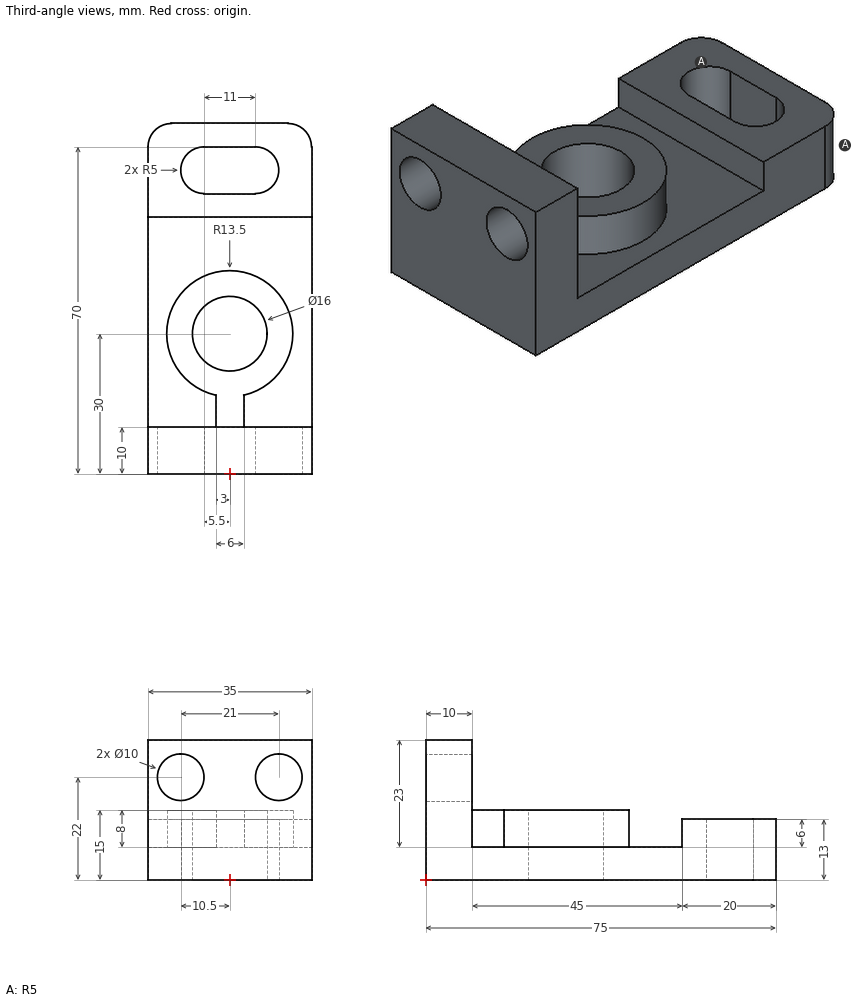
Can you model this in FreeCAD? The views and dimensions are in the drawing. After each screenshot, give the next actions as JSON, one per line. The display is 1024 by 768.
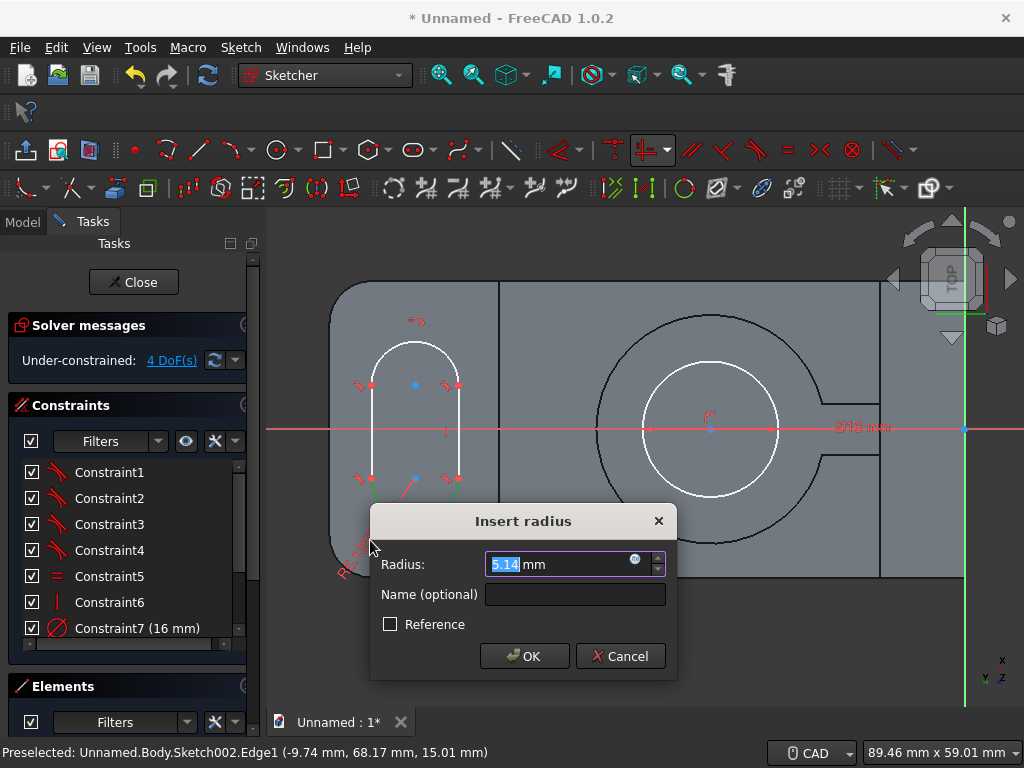
{"action": "type", "text": "5"}
{"action": "key", "text": "Return"}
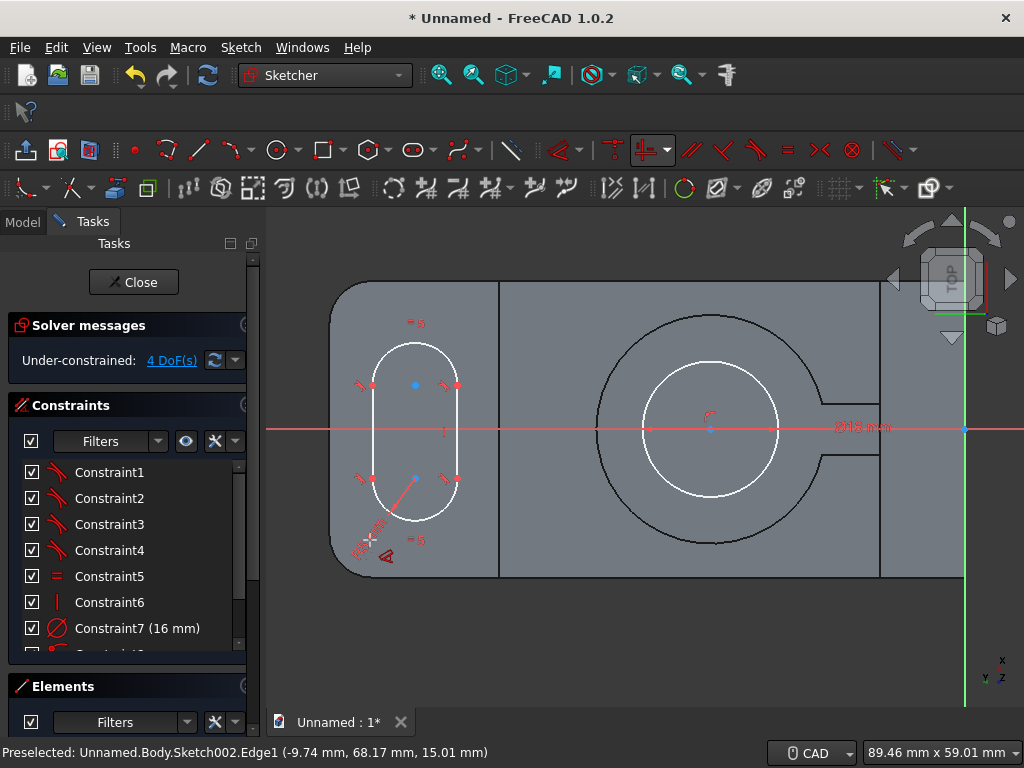
{"action": "left_click", "coordinate": [373, 450]}
{"action": "left_click", "coordinate": [339, 410]}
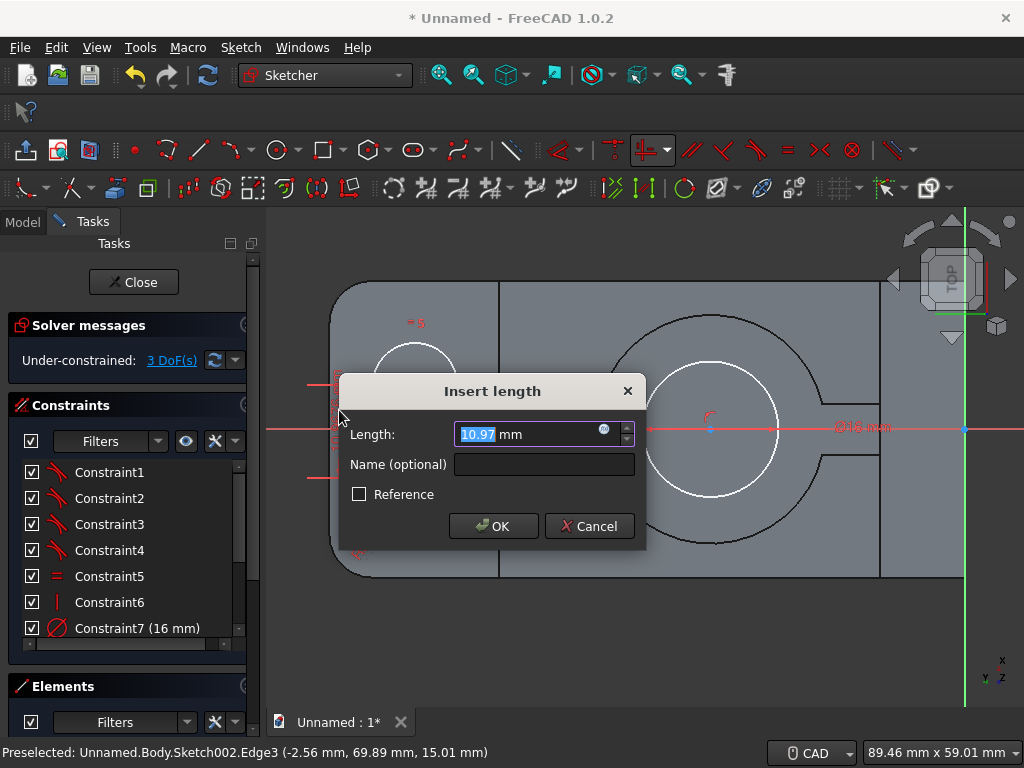
{"action": "type", "text": "11"}
{"action": "key", "text": "Return"}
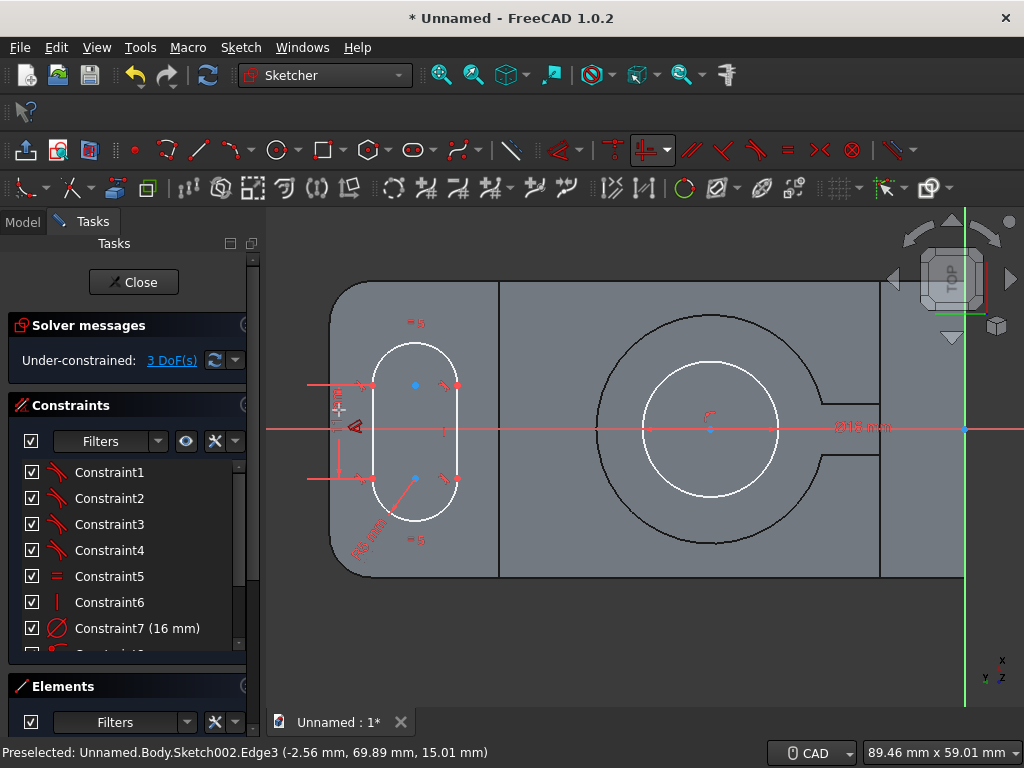
{"action": "left_click", "coordinate": [711, 429]}
{"action": "left_click", "coordinate": [785, 463]}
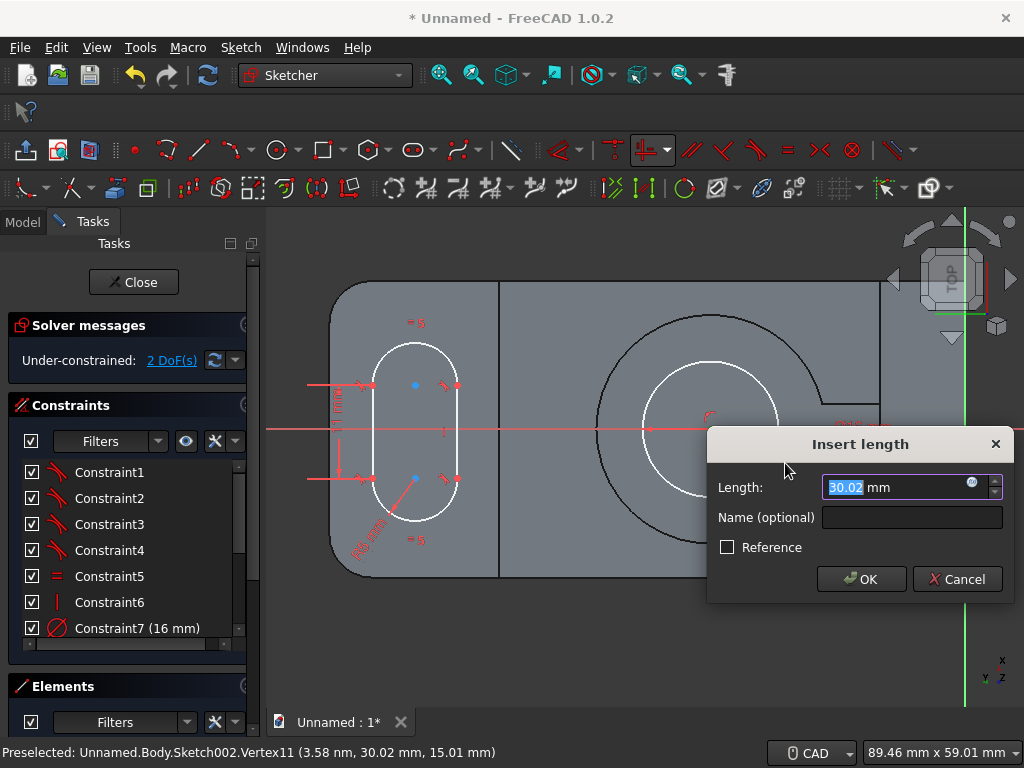
{"action": "type", "text": "30"}
{"action": "key", "text": "Return"}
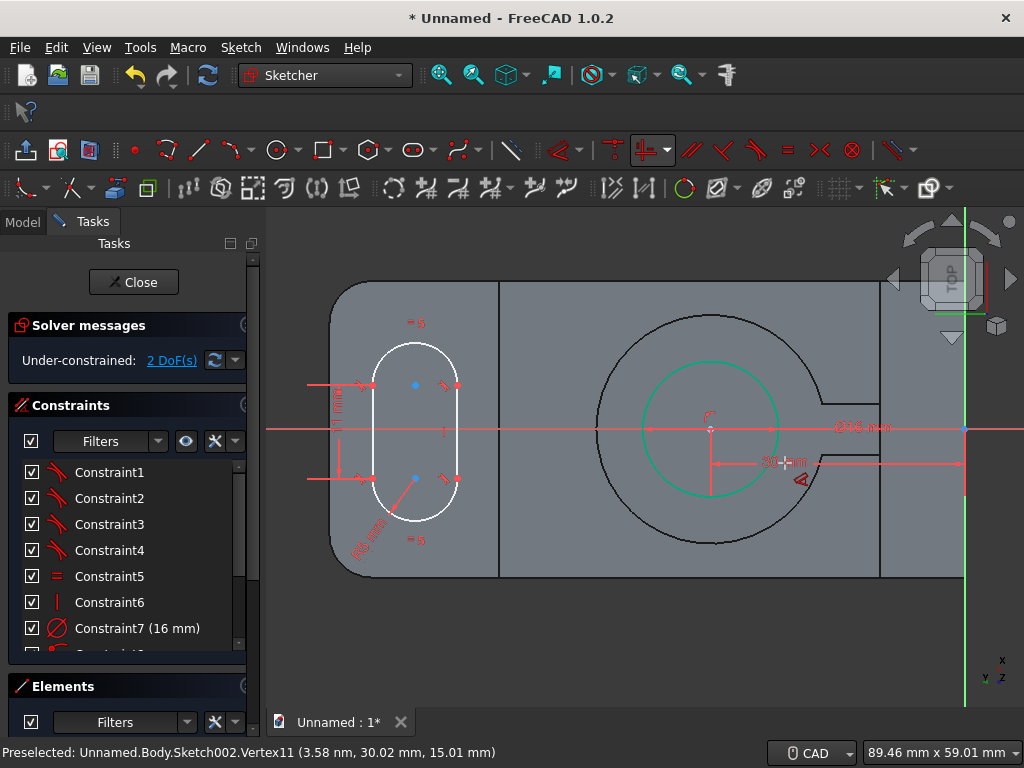
{"action": "left_click", "coordinate": [373, 479]}
{"action": "left_click", "coordinate": [616, 513]}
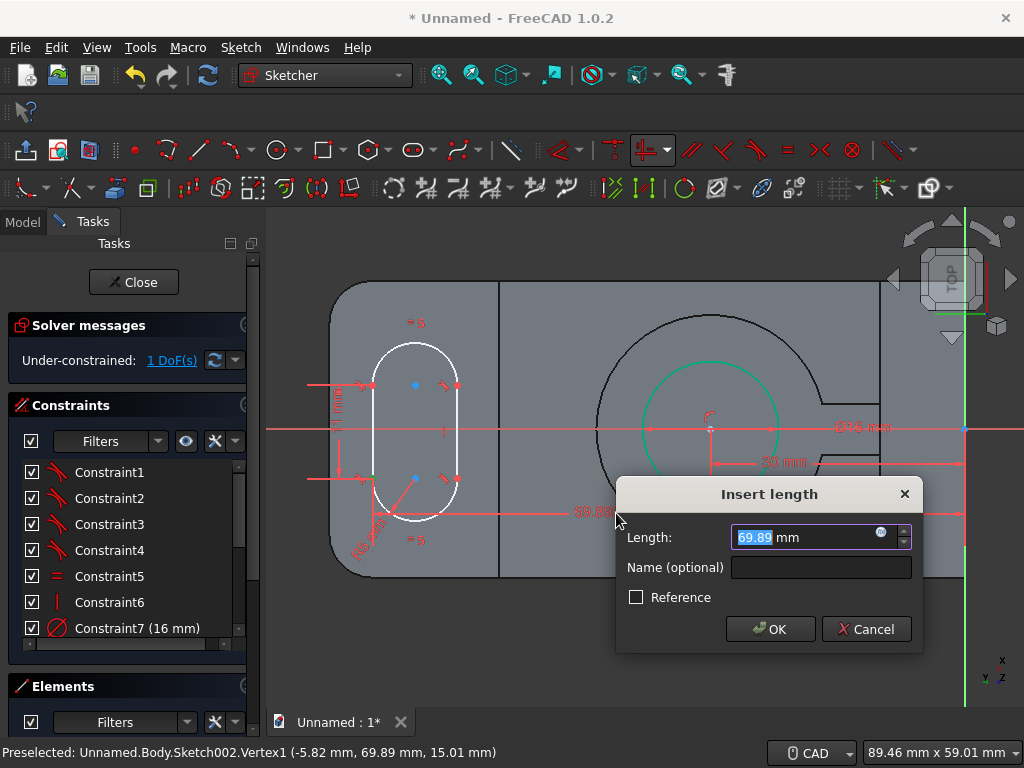
{"action": "type", "text": "70"}
{"action": "key", "text": "Return"}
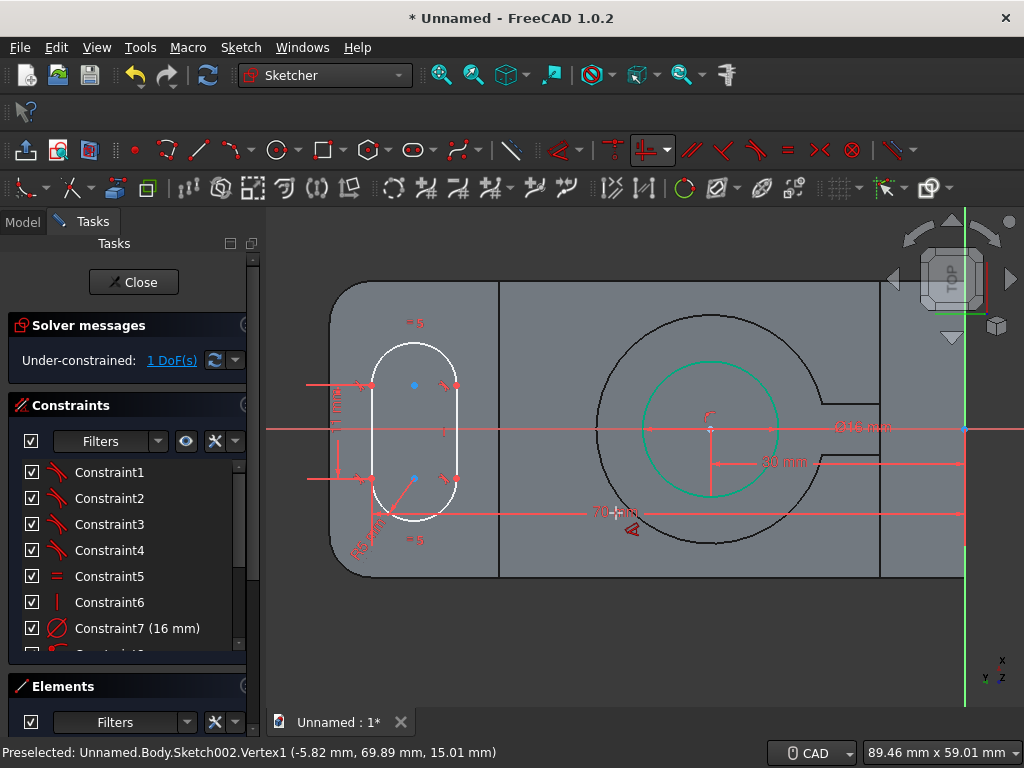
{"action": "left_click", "coordinate": [372, 479]}
{"action": "left_click", "coordinate": [338, 454]}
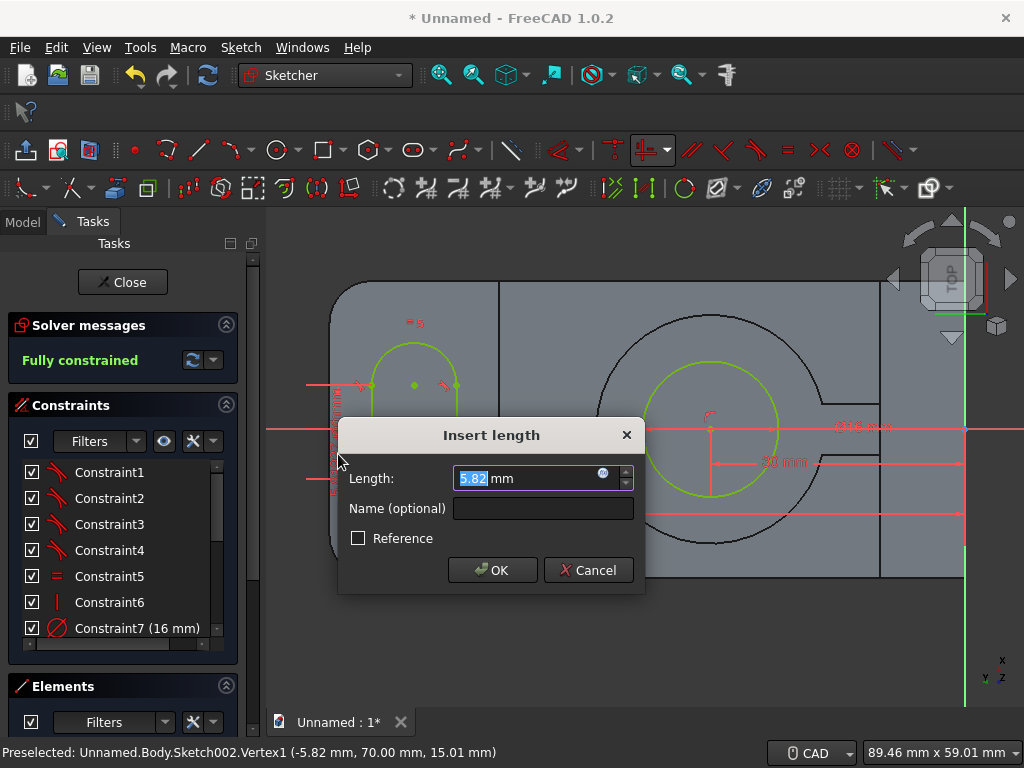
{"action": "type", "text": "5.5"}
{"action": "key", "text": "Return"}
{"action": "key", "text": "Escape"}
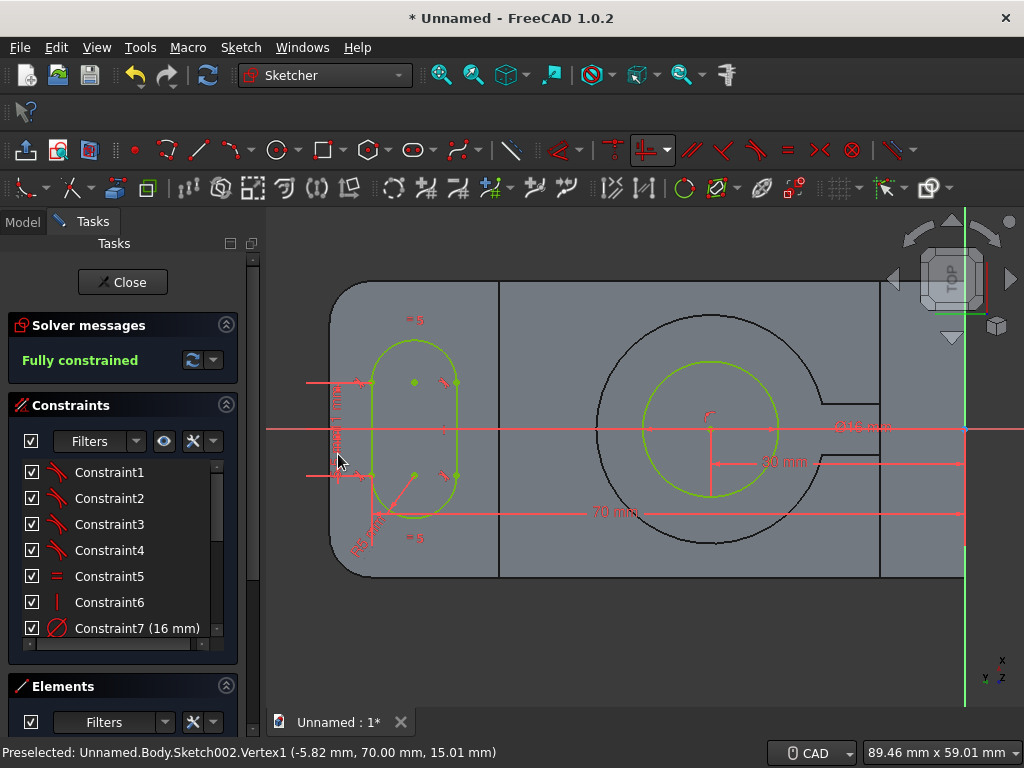
{"action": "left_click", "coordinate": [123, 282]}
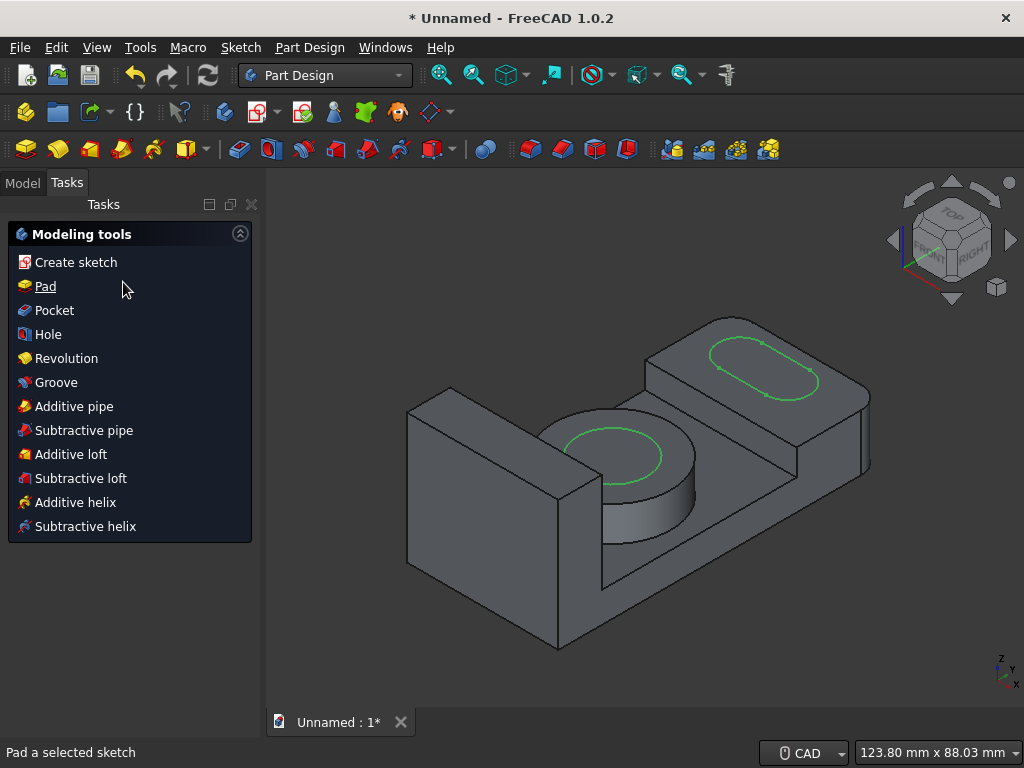
{"action": "left_click", "coordinate": [240, 150]}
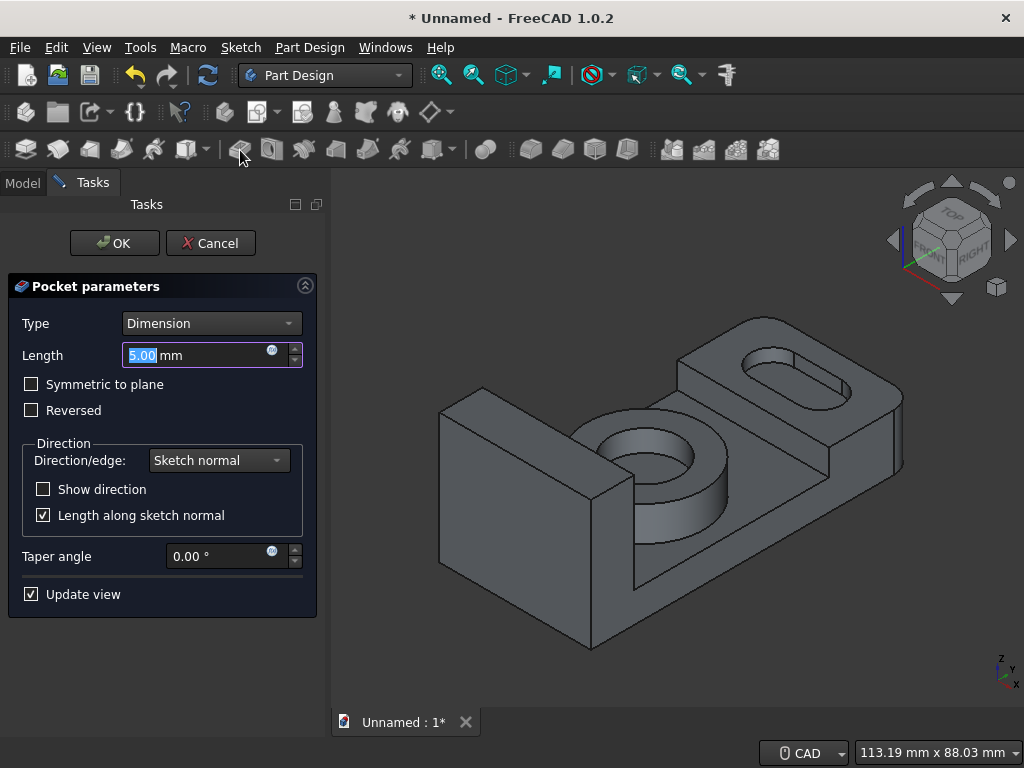
{"action": "type", "text": "15"}
{"action": "key", "text": "Tab"}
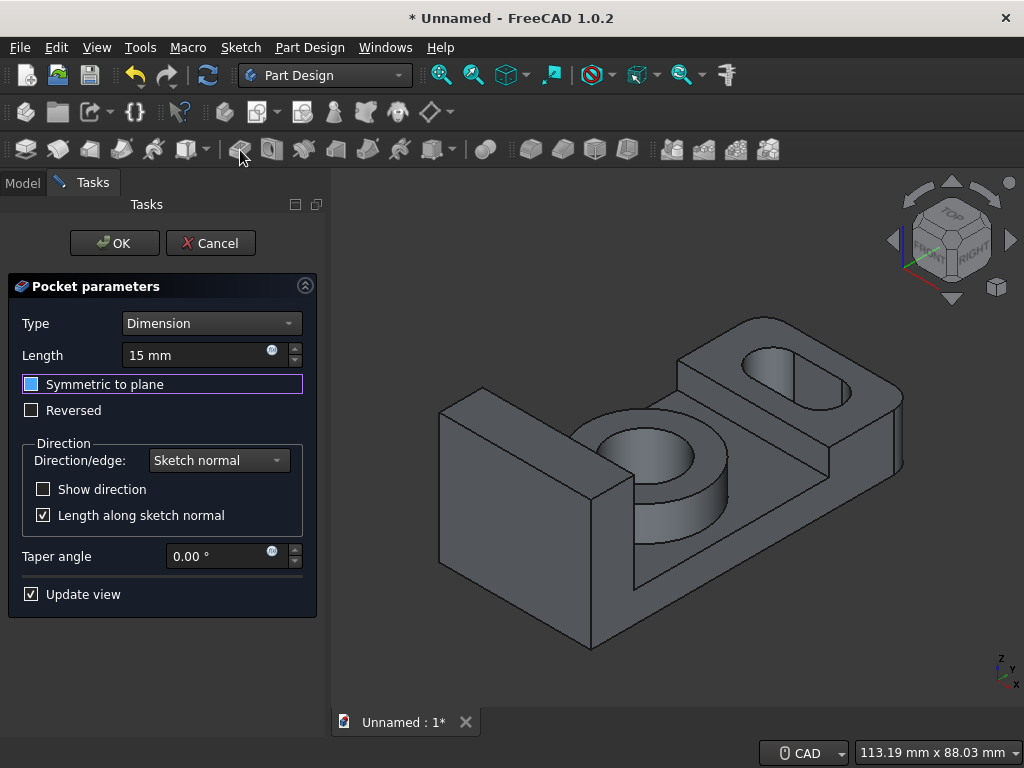
{"action": "left_click", "coordinate": [115, 243]}